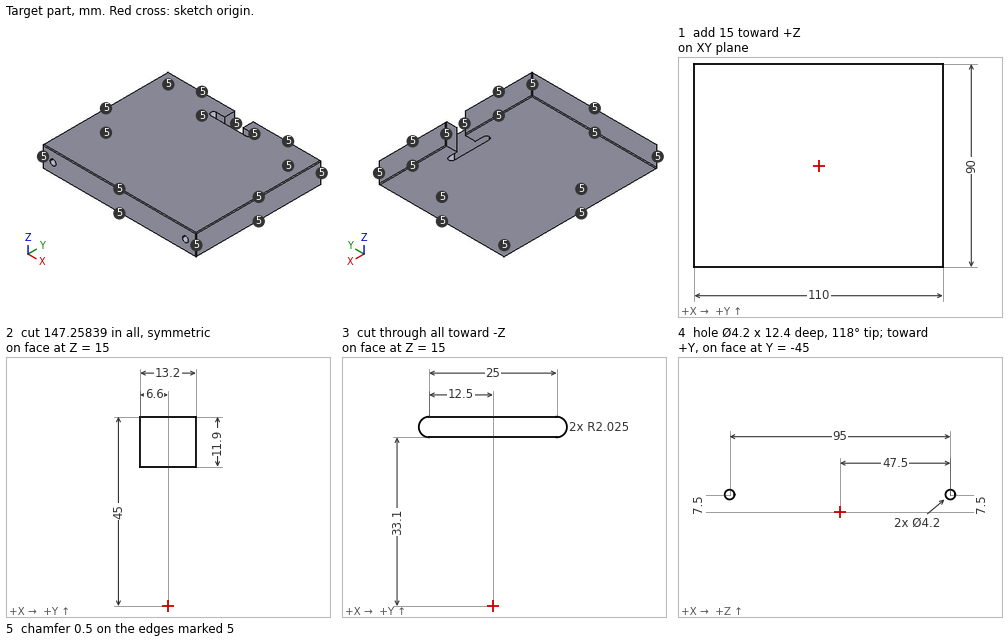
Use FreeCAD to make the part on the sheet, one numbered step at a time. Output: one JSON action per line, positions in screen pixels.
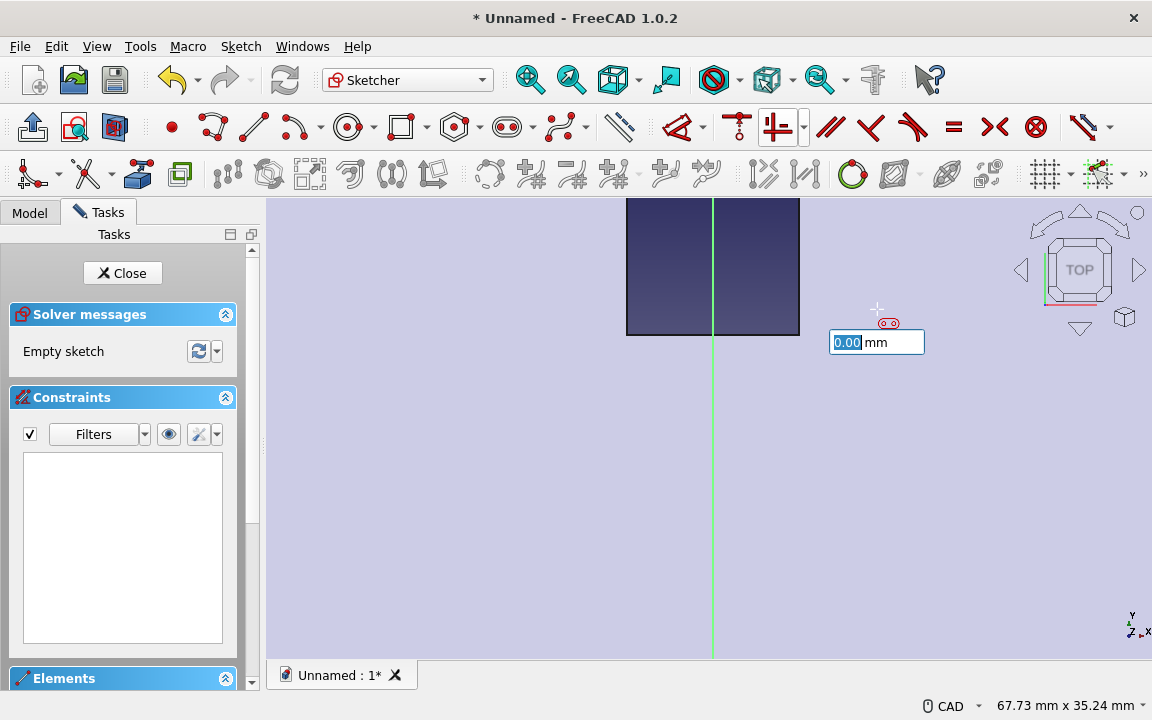
{"action": "left_click", "coordinate": [762, 282]}
{"action": "key", "text": "Escape"}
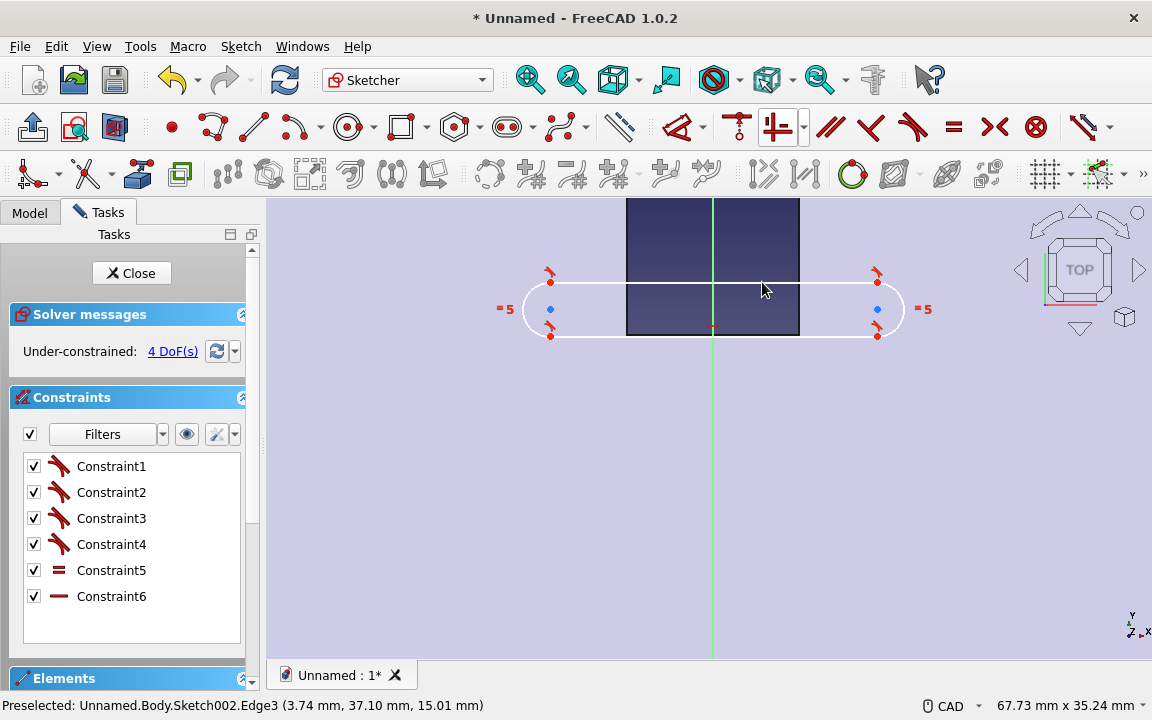
{"action": "left_click", "coordinate": [676, 128]}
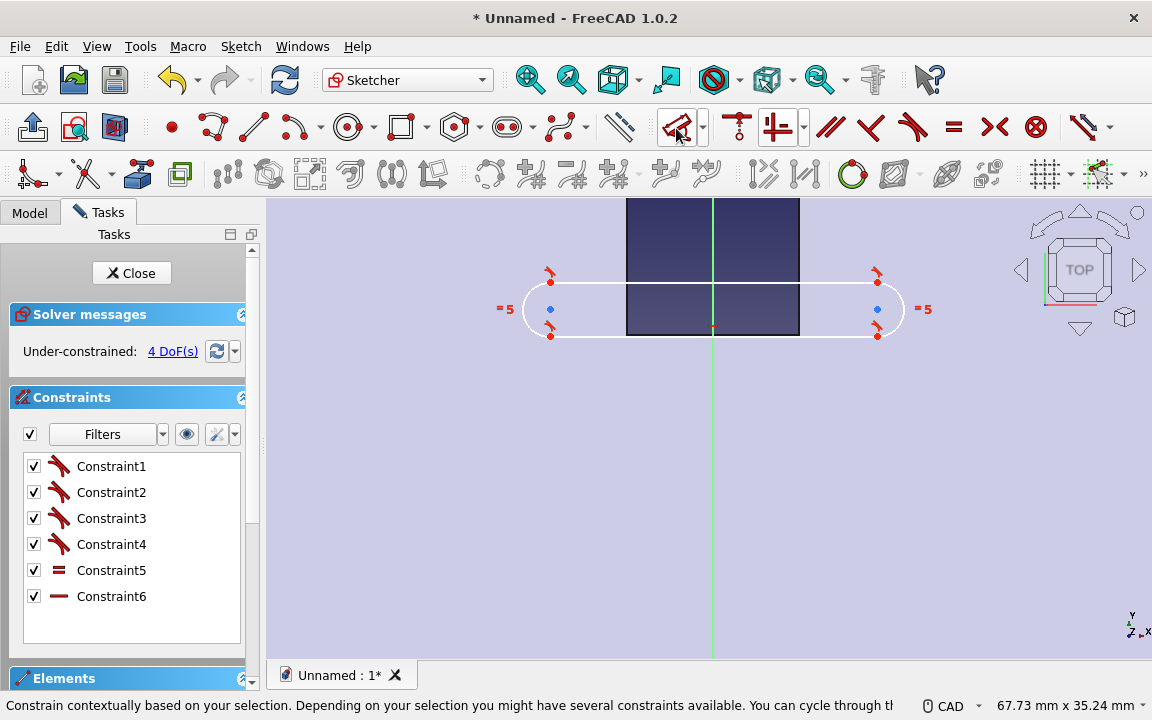
{"action": "scroll", "coordinate": [528, 294], "scroll_direction": "up", "scroll_amount": 3}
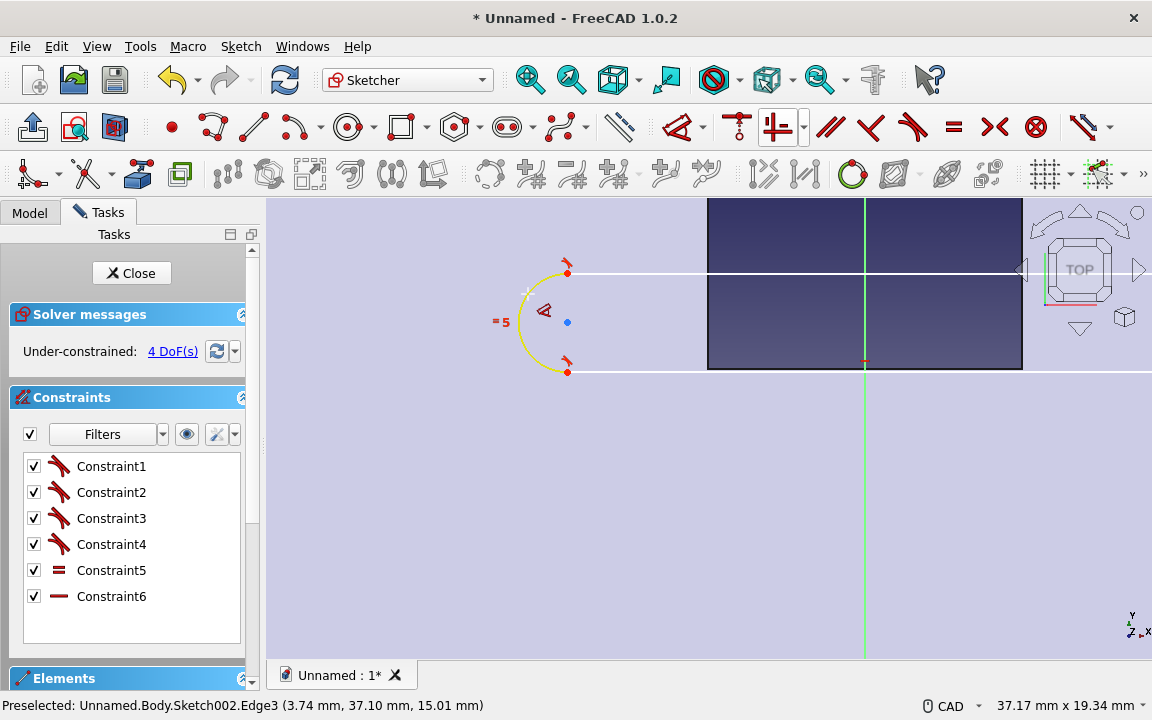
{"action": "left_click", "coordinate": [528, 294]}
{"action": "left_click", "coordinate": [502, 275]}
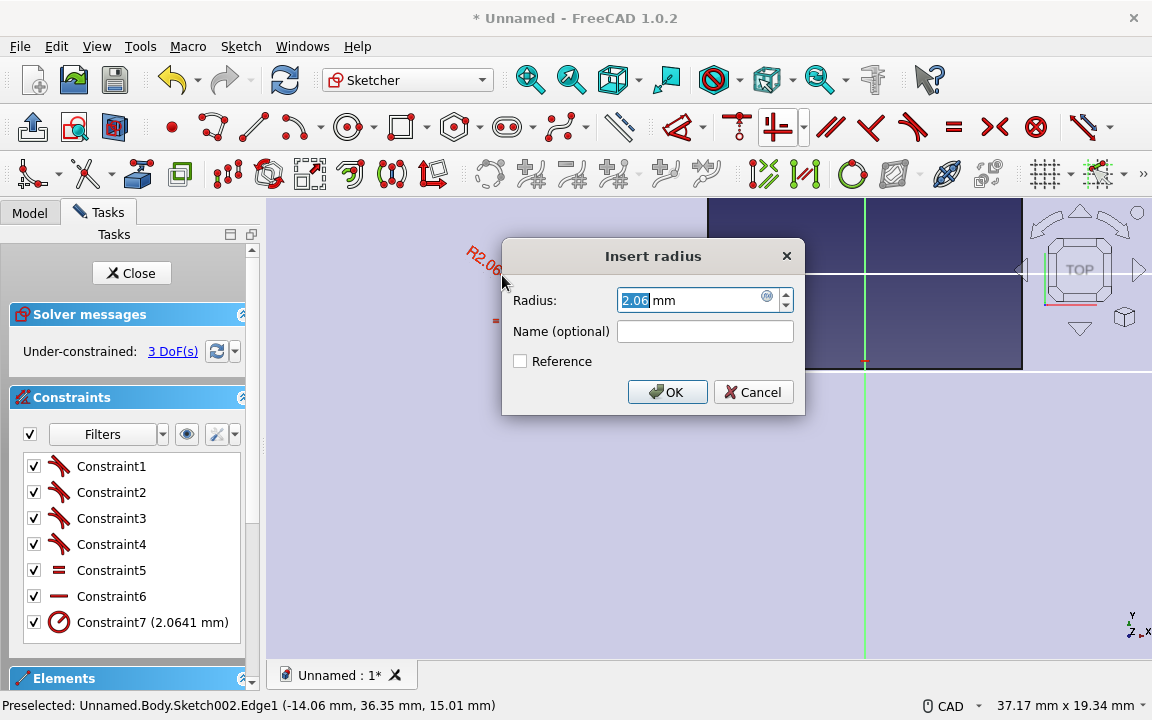
{"action": "type", "text": "2.025"}
{"action": "key", "text": "Return"}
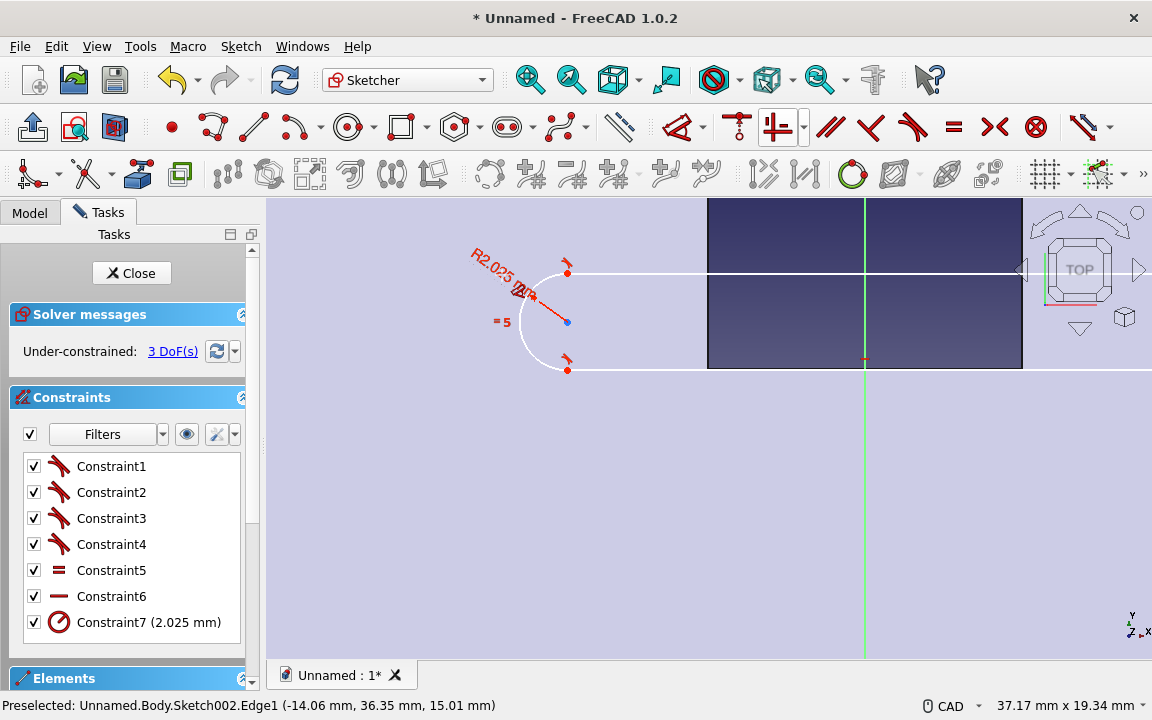
{"action": "left_click", "coordinate": [747, 274]}
{"action": "left_click", "coordinate": [777, 240]}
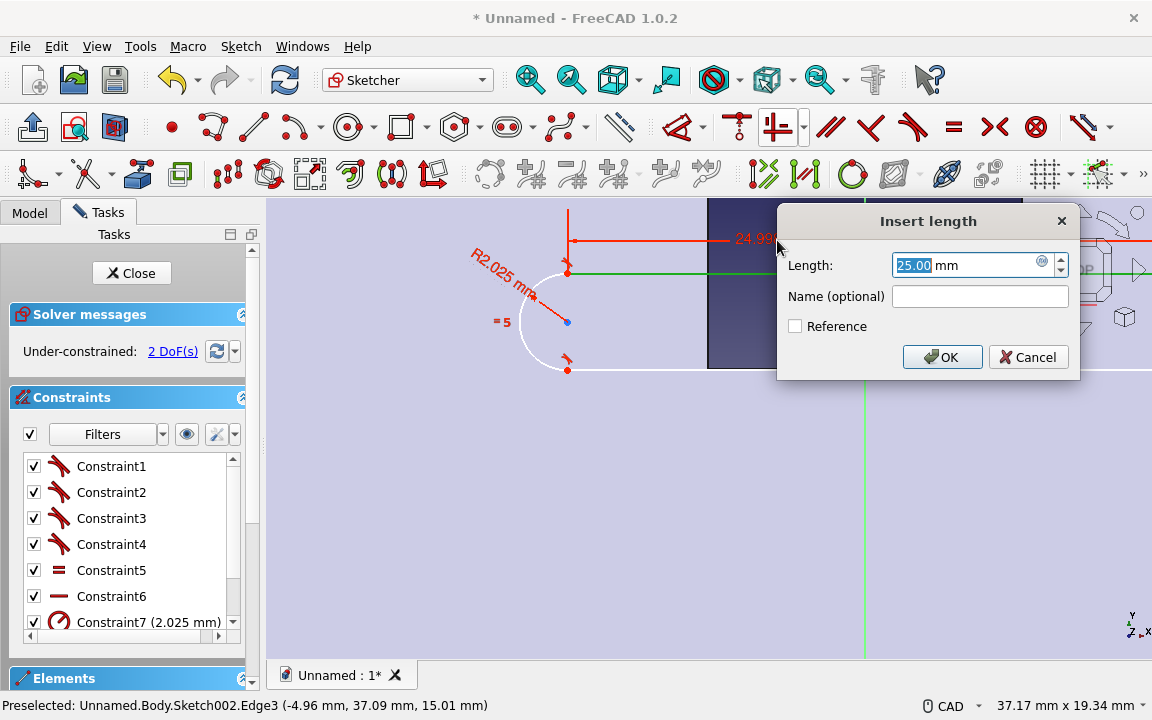
{"action": "type", "text": "25"}
{"action": "key", "text": "Return"}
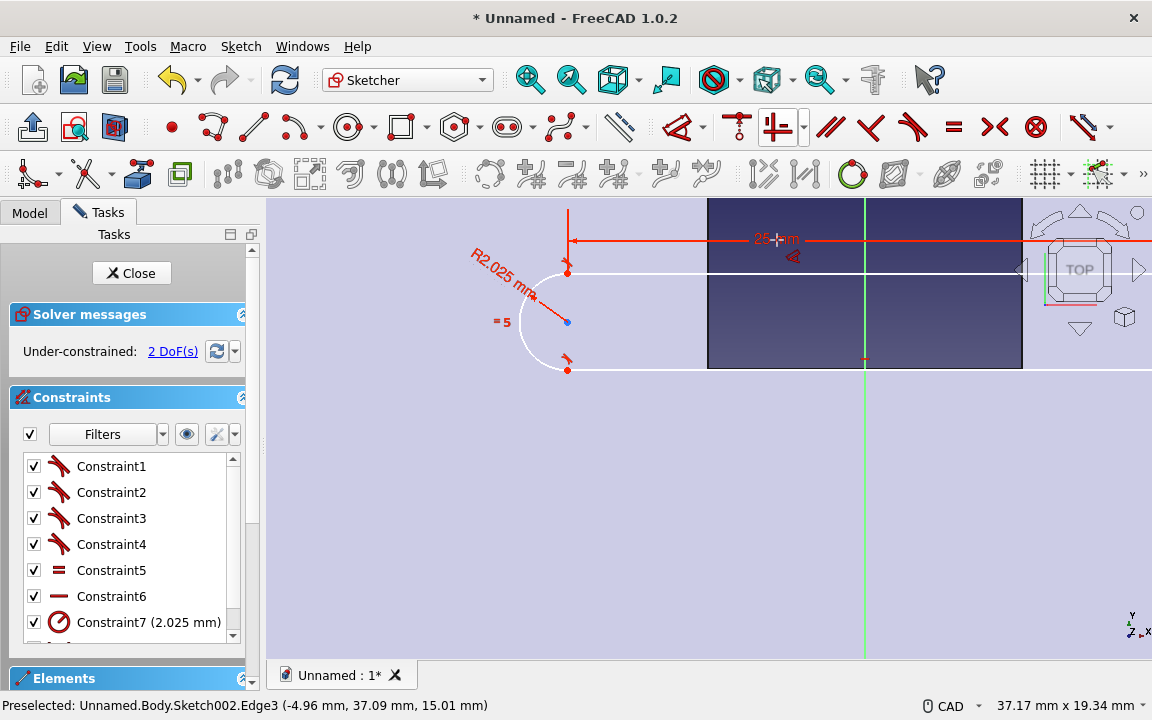
{"action": "left_click", "coordinate": [568, 274]}
{"action": "left_click", "coordinate": [648, 240]}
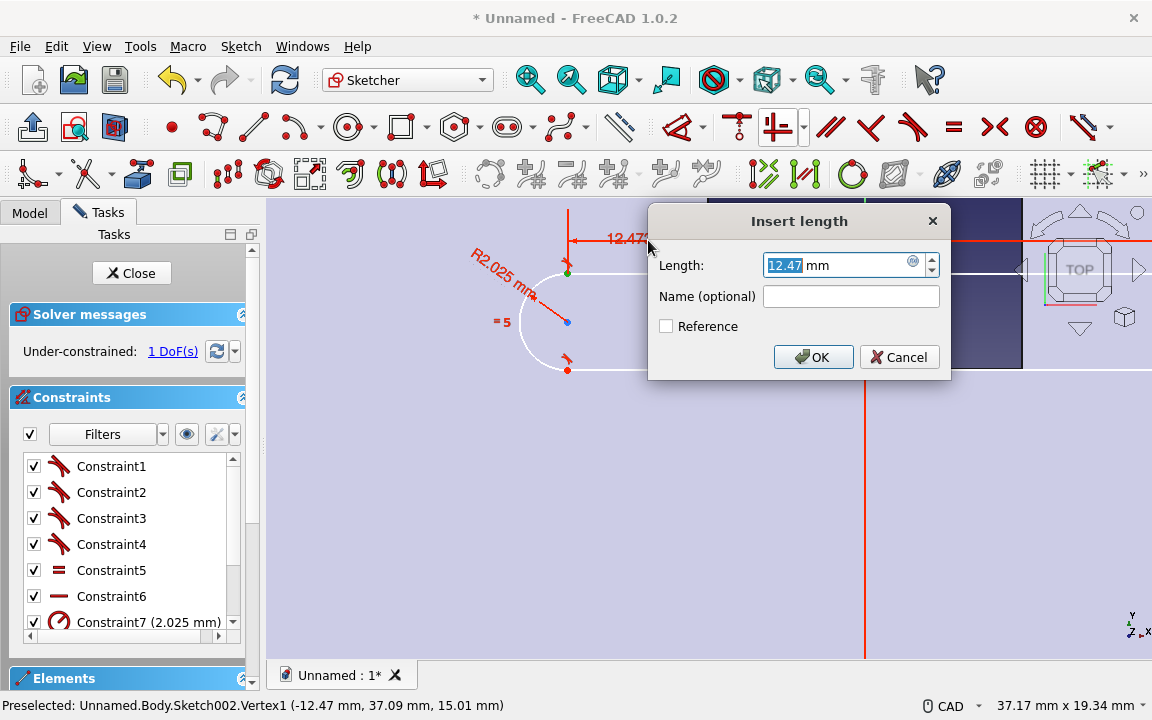
{"action": "type", "text": "12.5"}
{"action": "key", "text": "Return"}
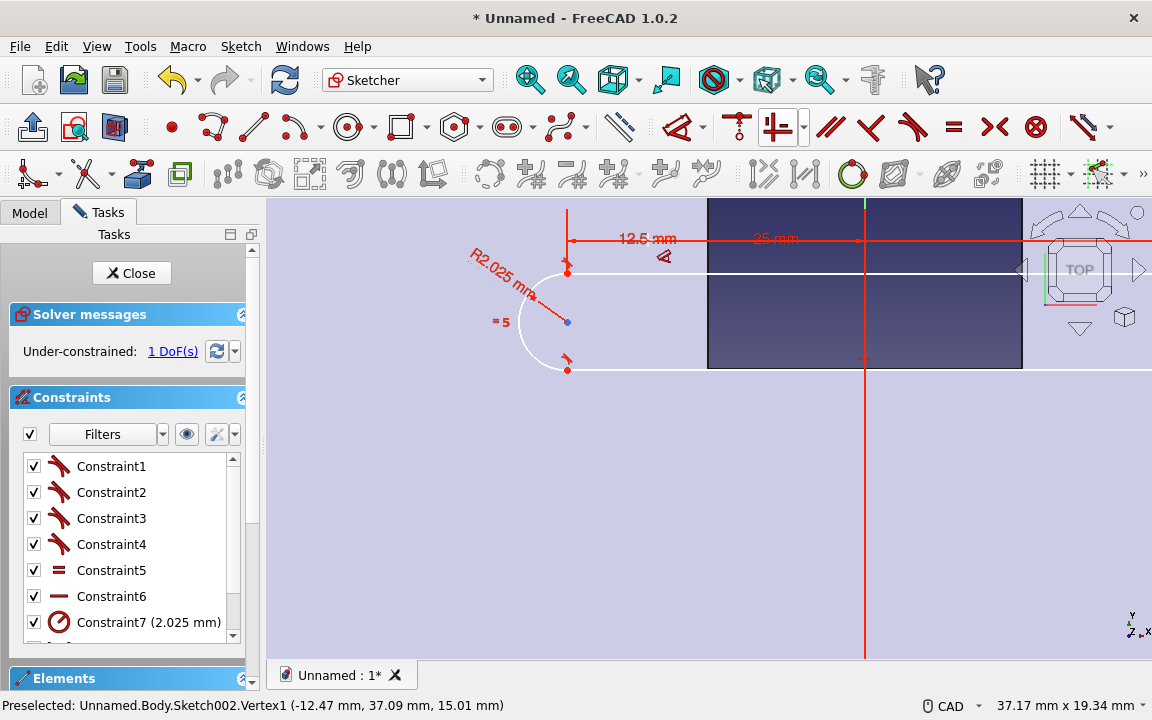
{"action": "left_click", "coordinate": [567, 370]}
{"action": "left_click", "coordinate": [533, 501]}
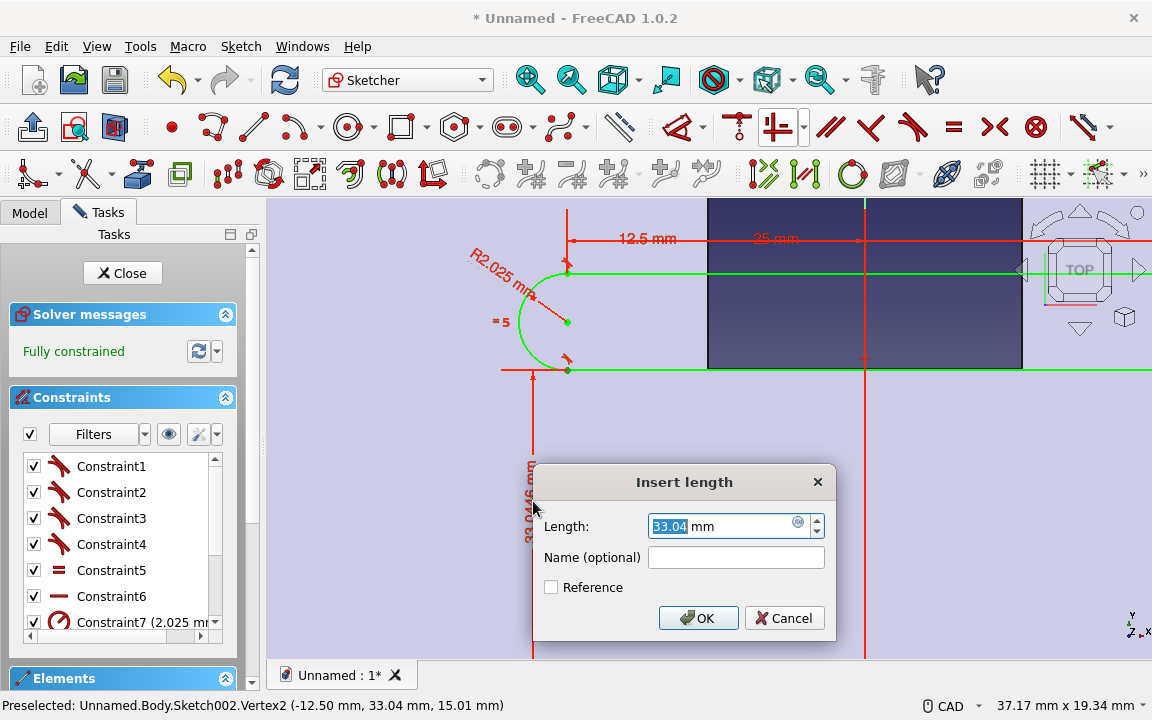
{"action": "type", "text": "33.1"}
{"action": "key", "text": "Return"}
{"action": "key", "text": "Escape"}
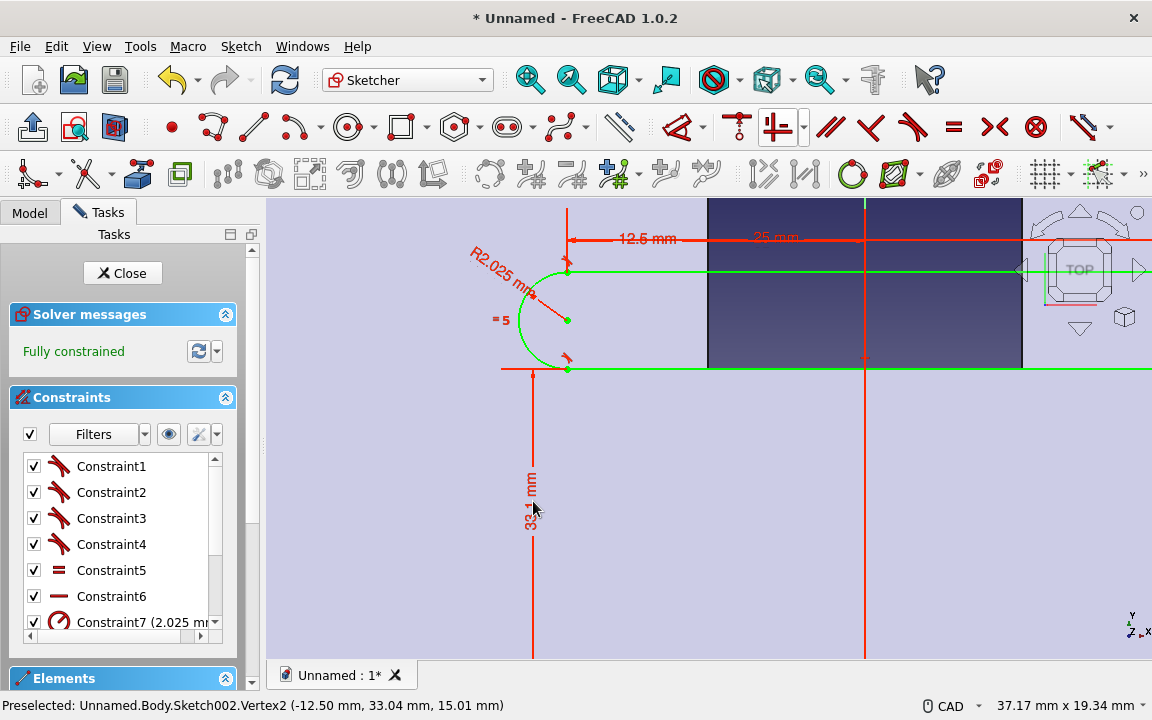
{"action": "left_click", "coordinate": [123, 273]}